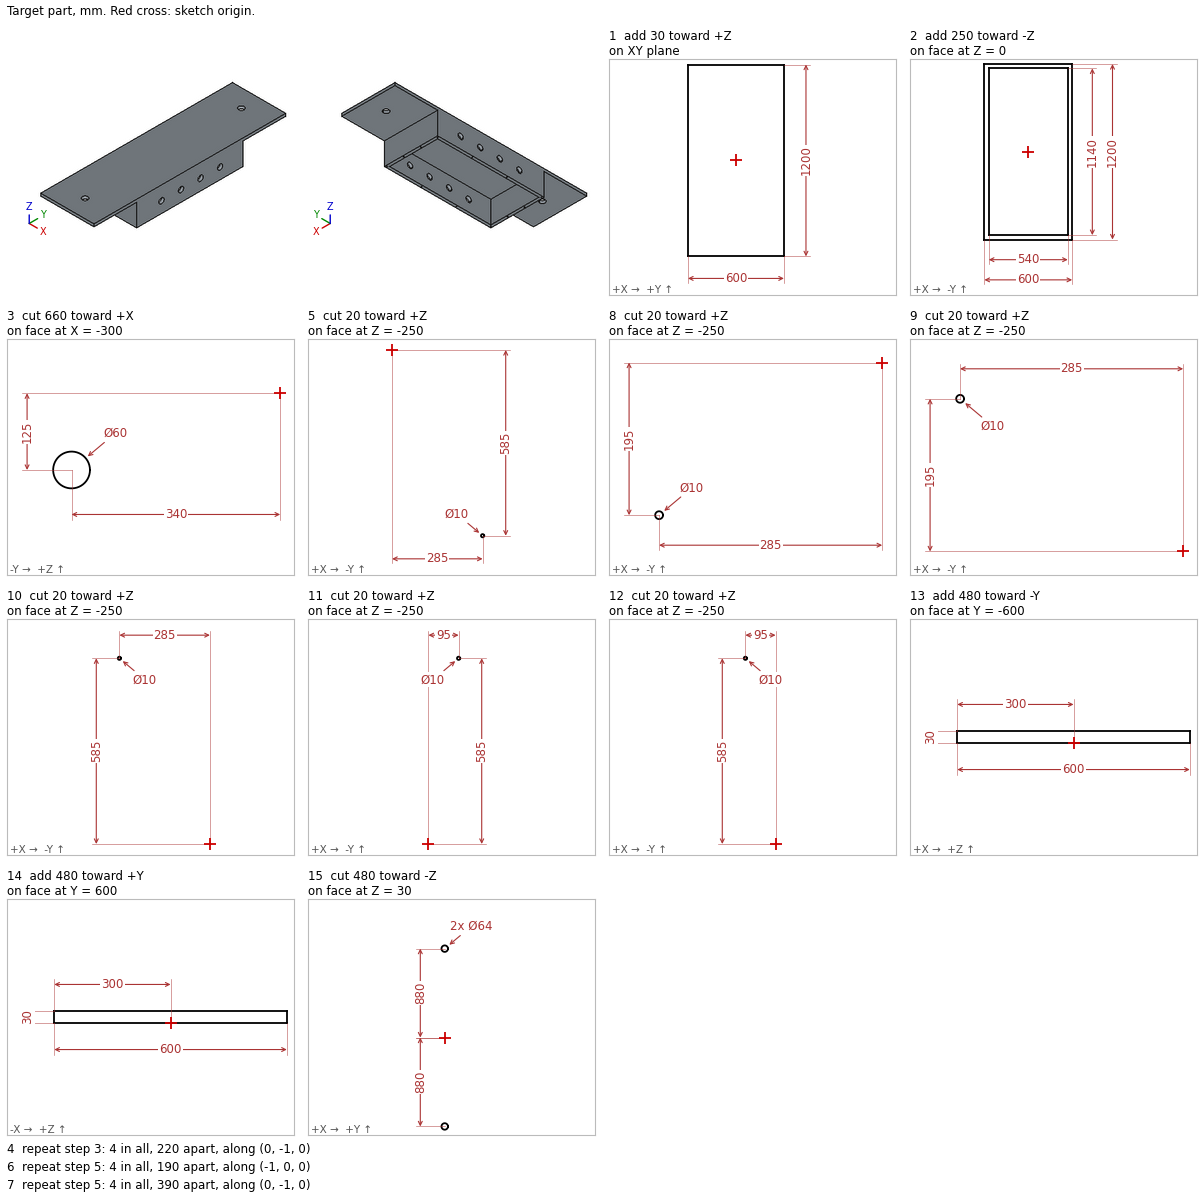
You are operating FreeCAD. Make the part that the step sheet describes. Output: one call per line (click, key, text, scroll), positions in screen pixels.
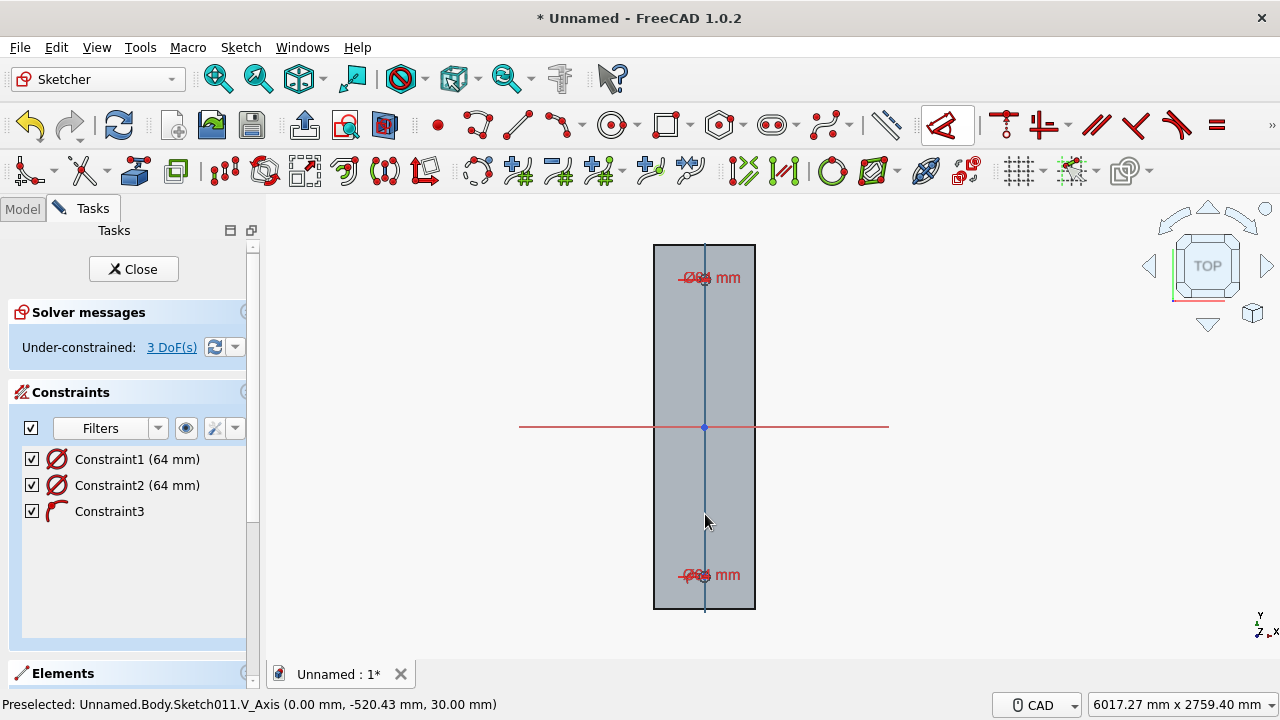
click(1004, 126)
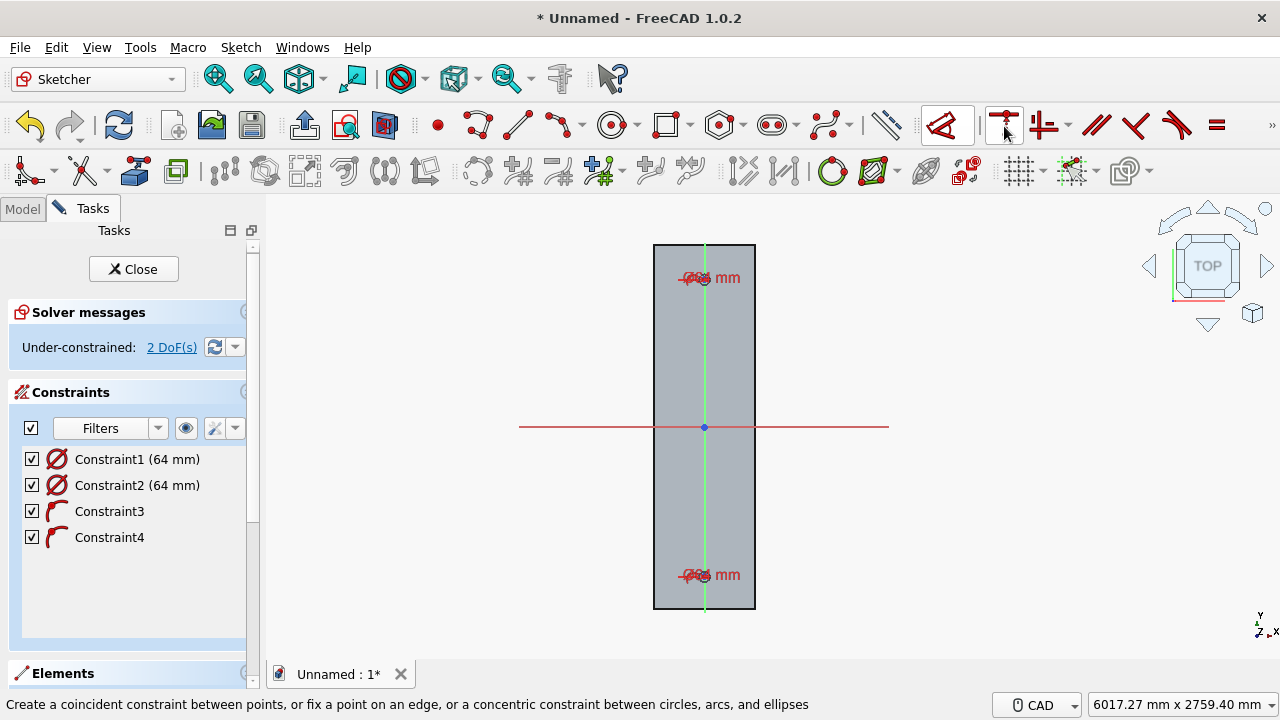
click(705, 280)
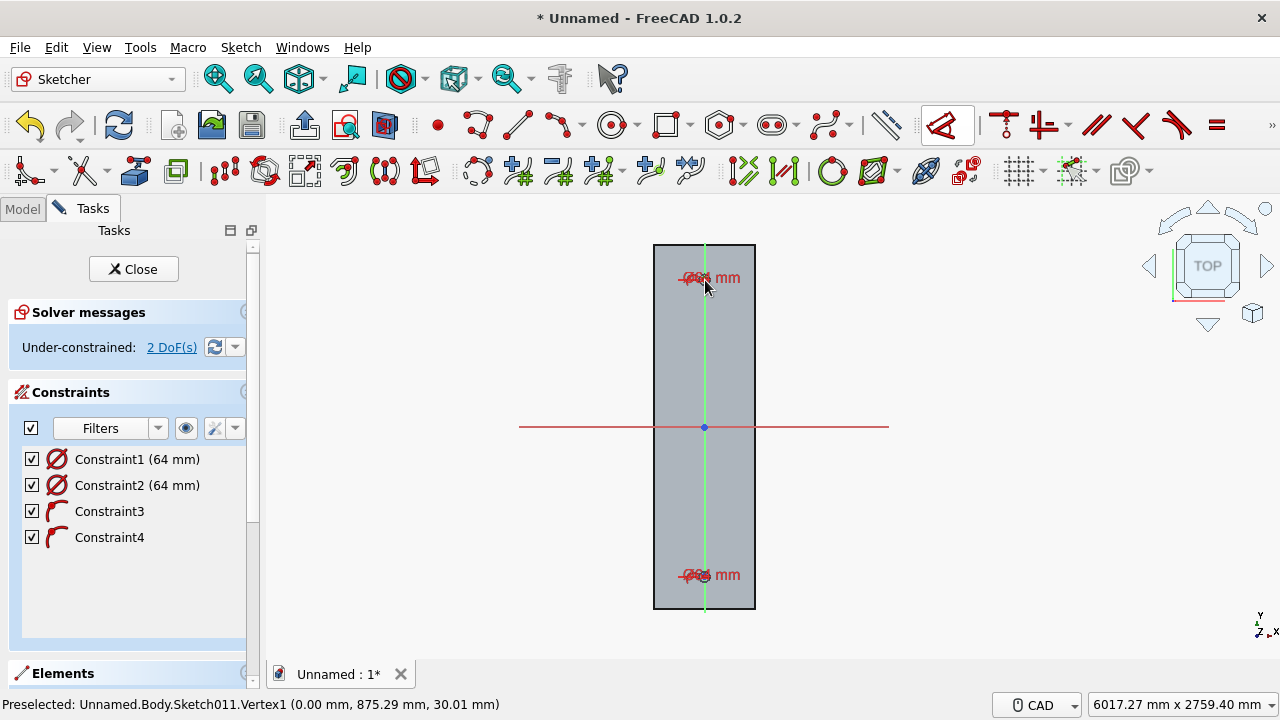
click(968, 126)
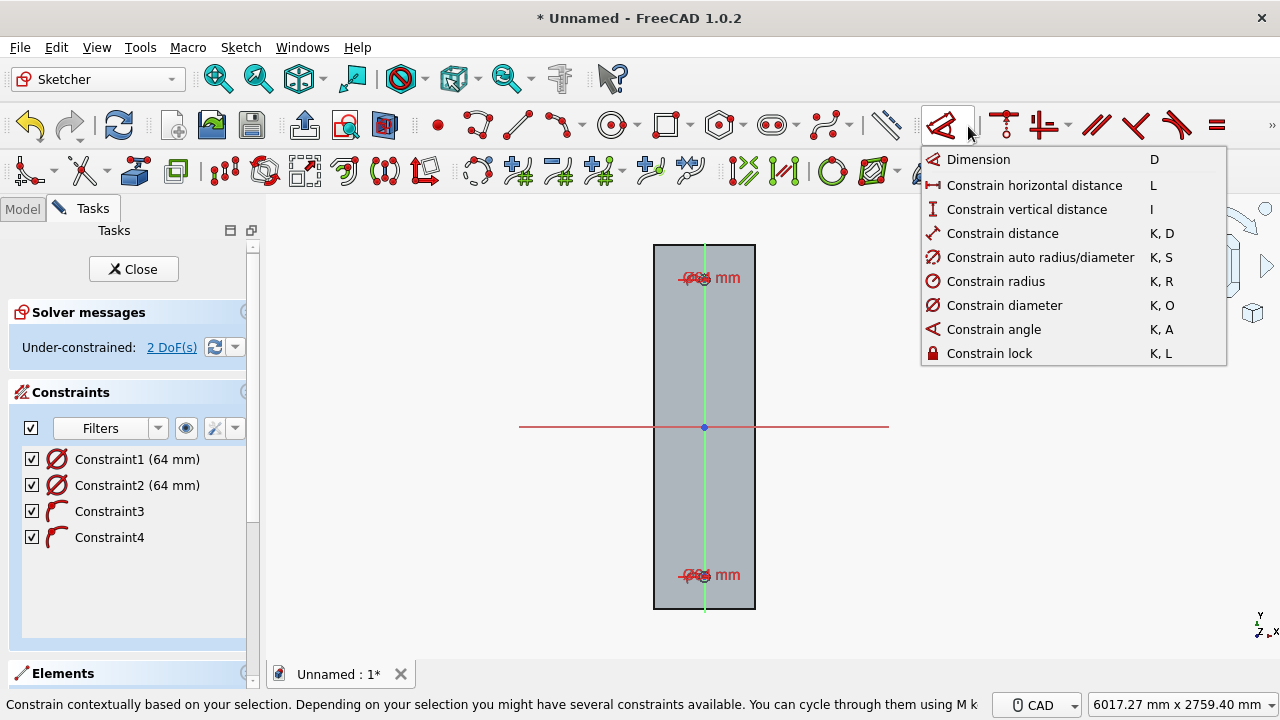
click(1074, 209)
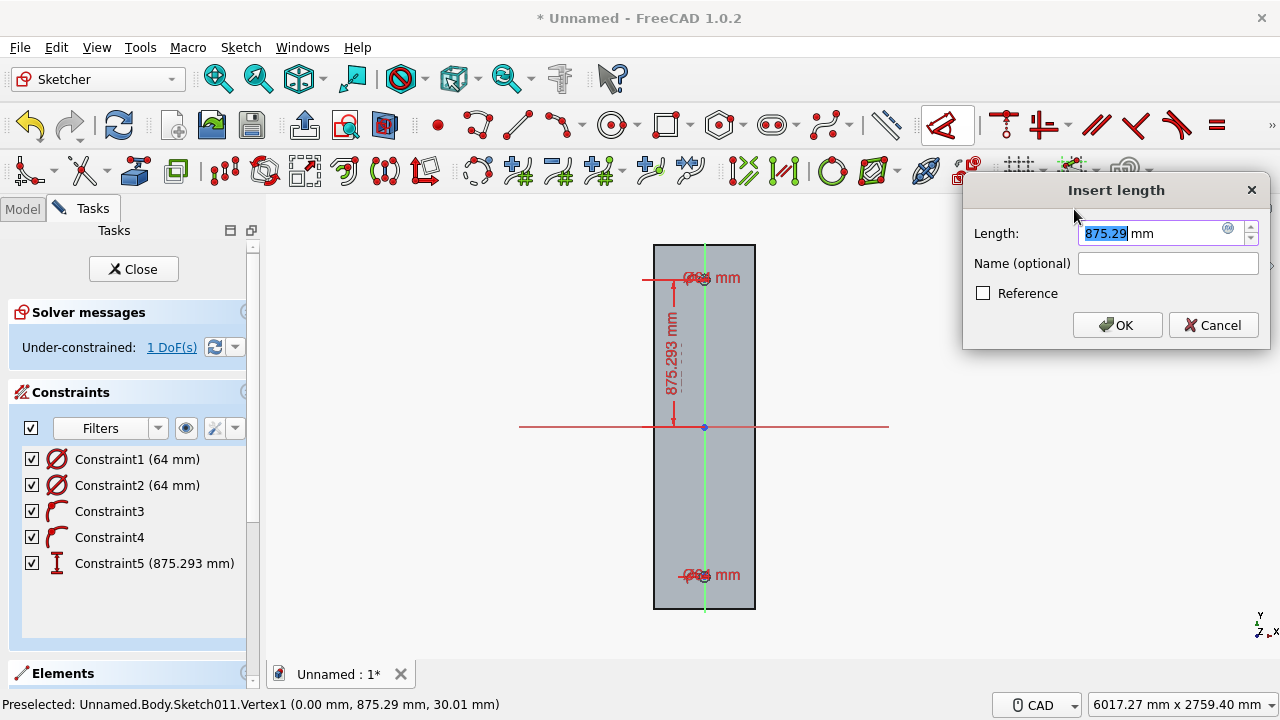
text(880)
key(Return)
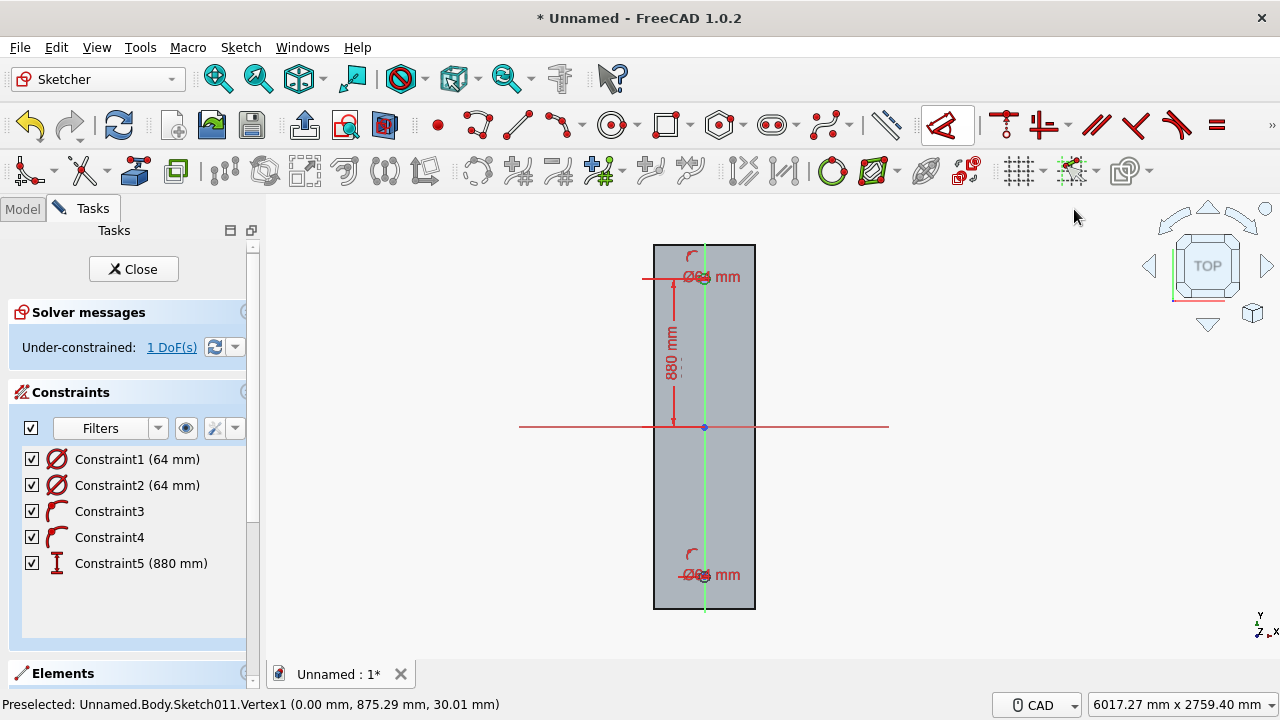
click(705, 577)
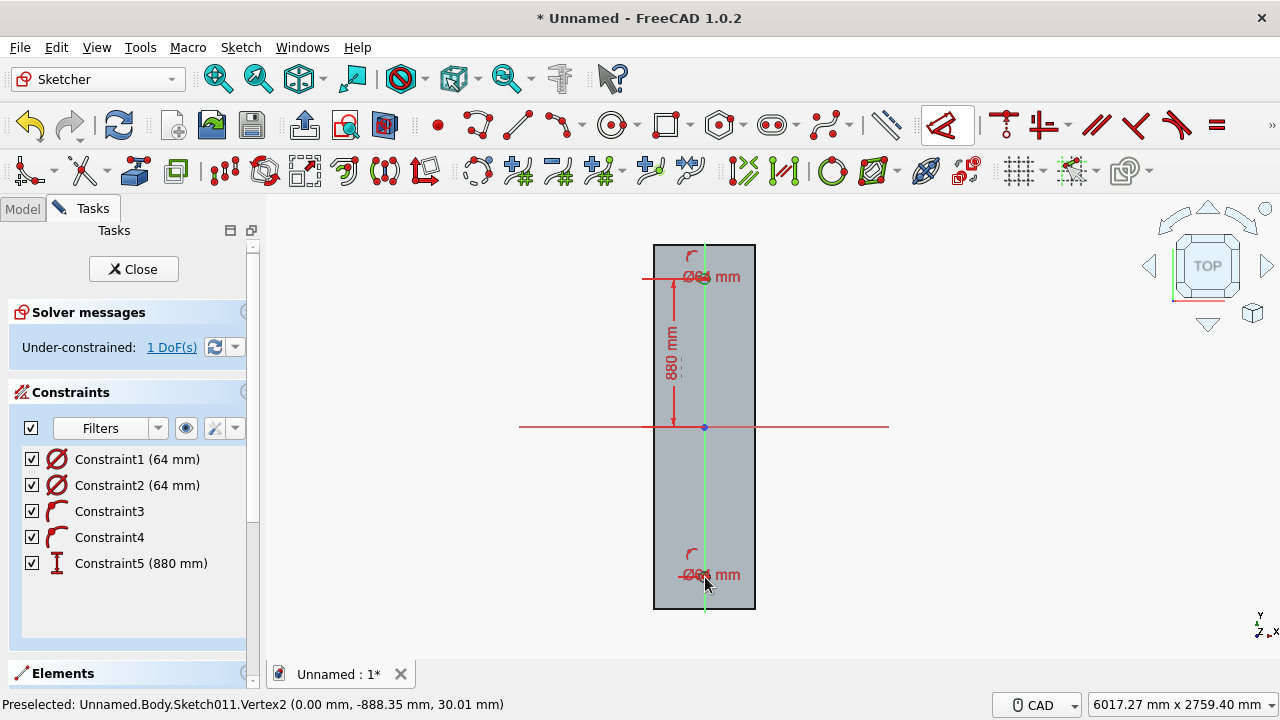
key(i)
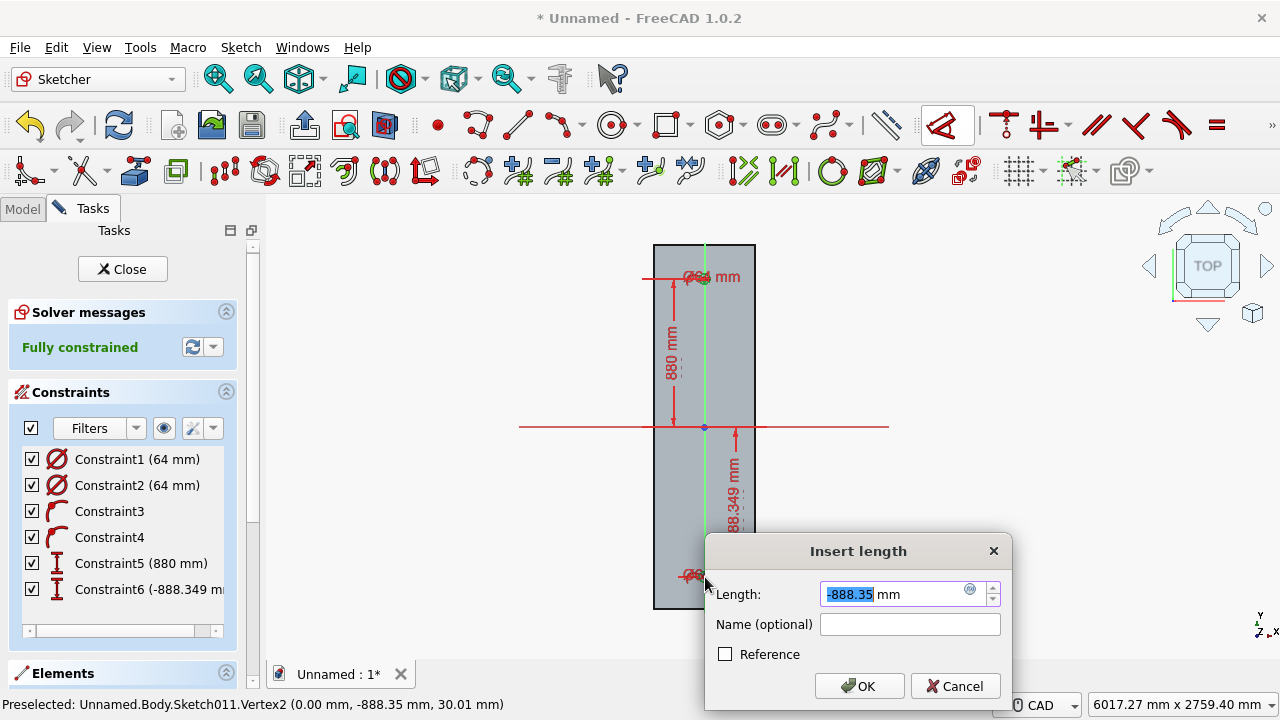
text(-880)
key(Return)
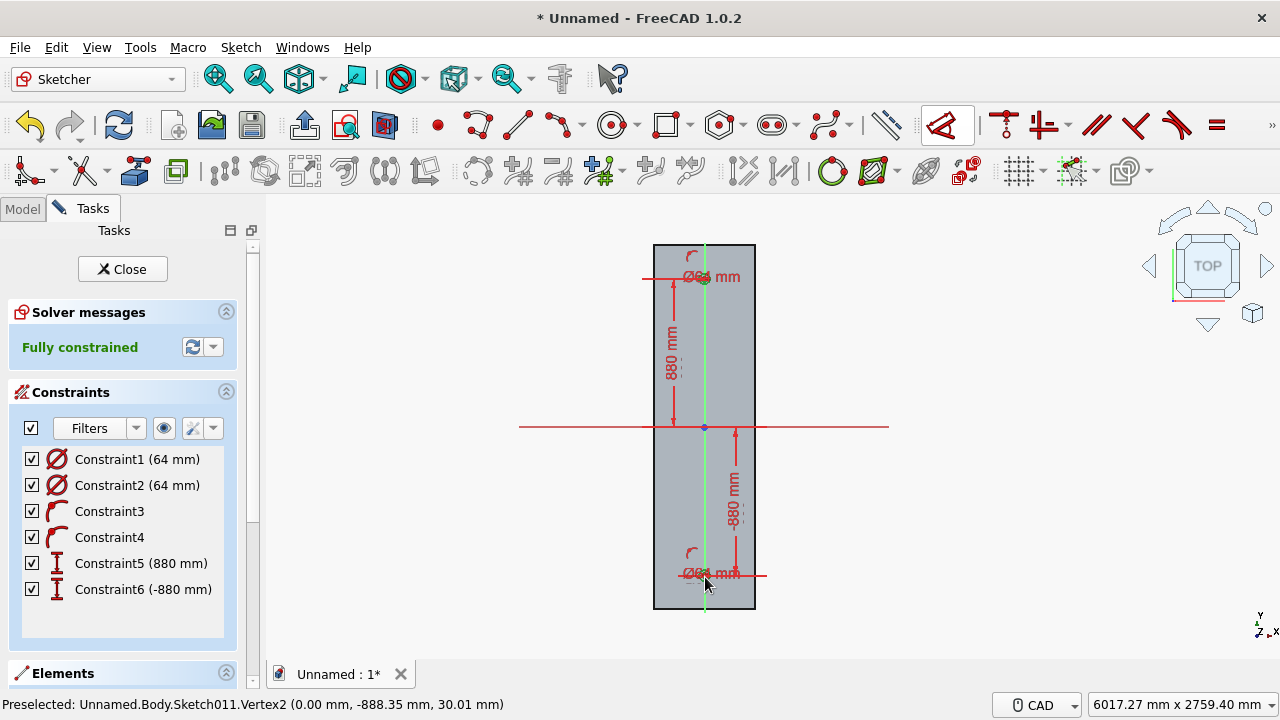
click(123, 269)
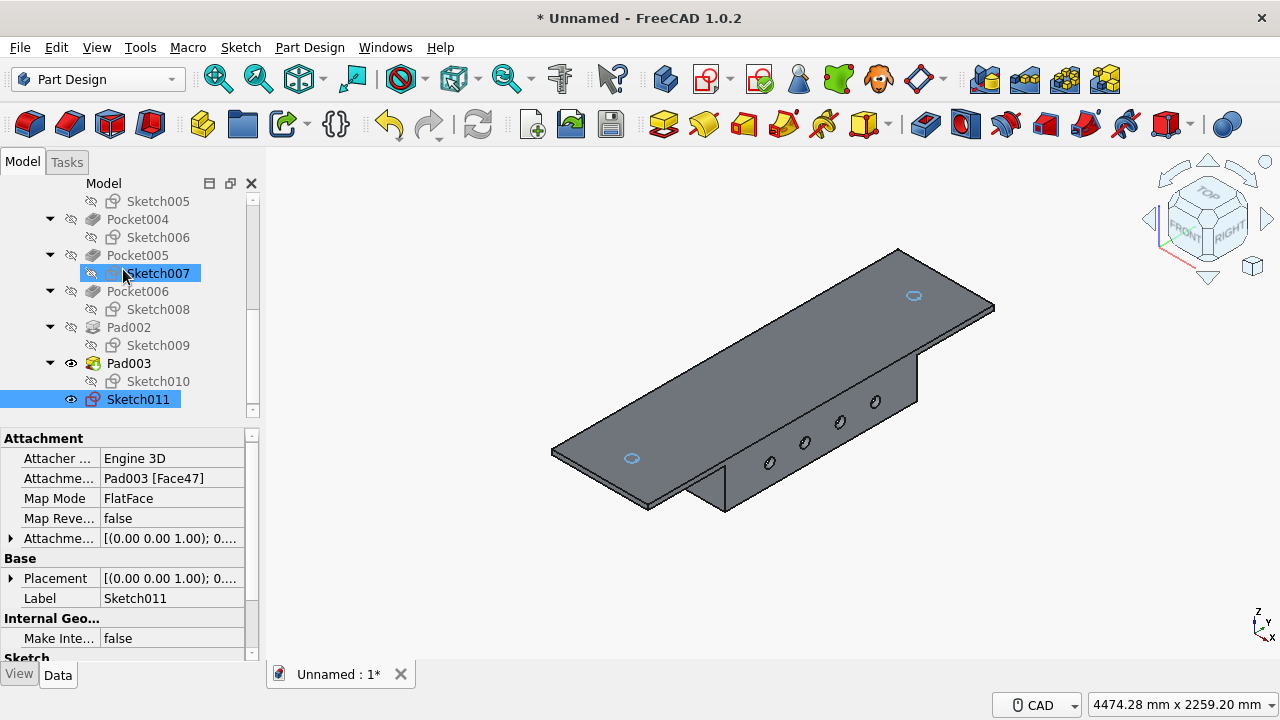
click(926, 124)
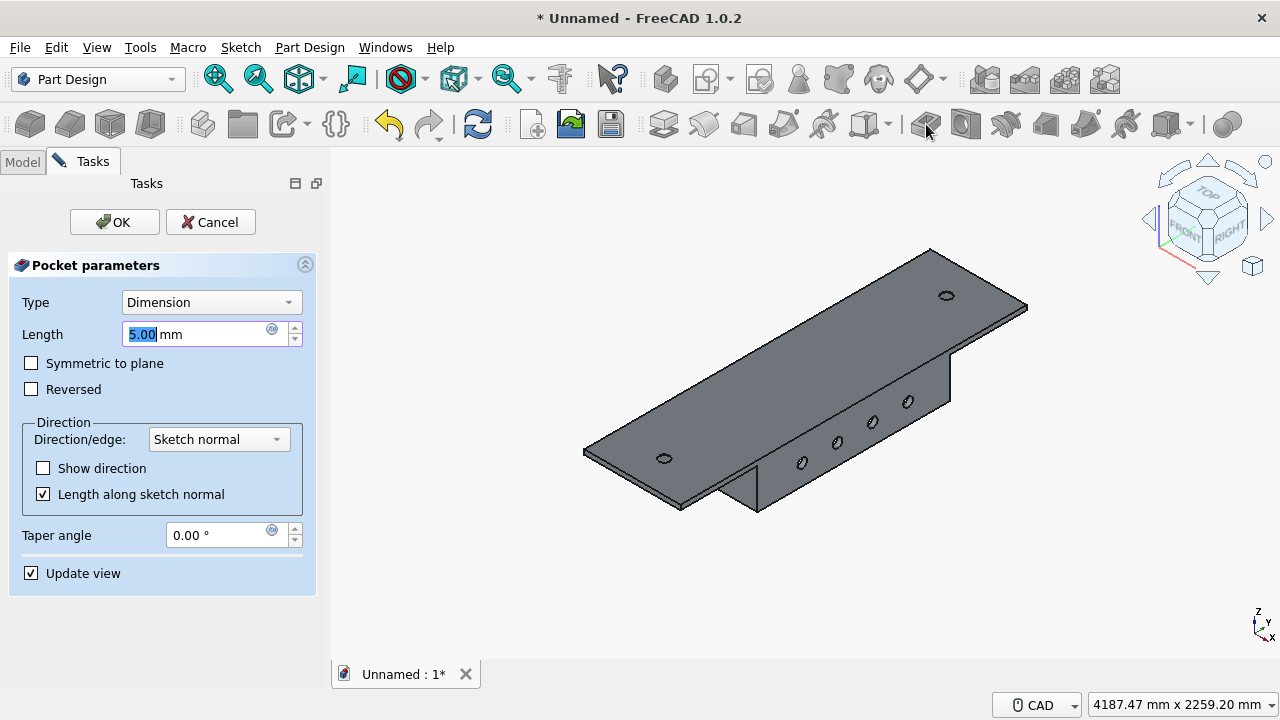
text(480)
key(Tab)